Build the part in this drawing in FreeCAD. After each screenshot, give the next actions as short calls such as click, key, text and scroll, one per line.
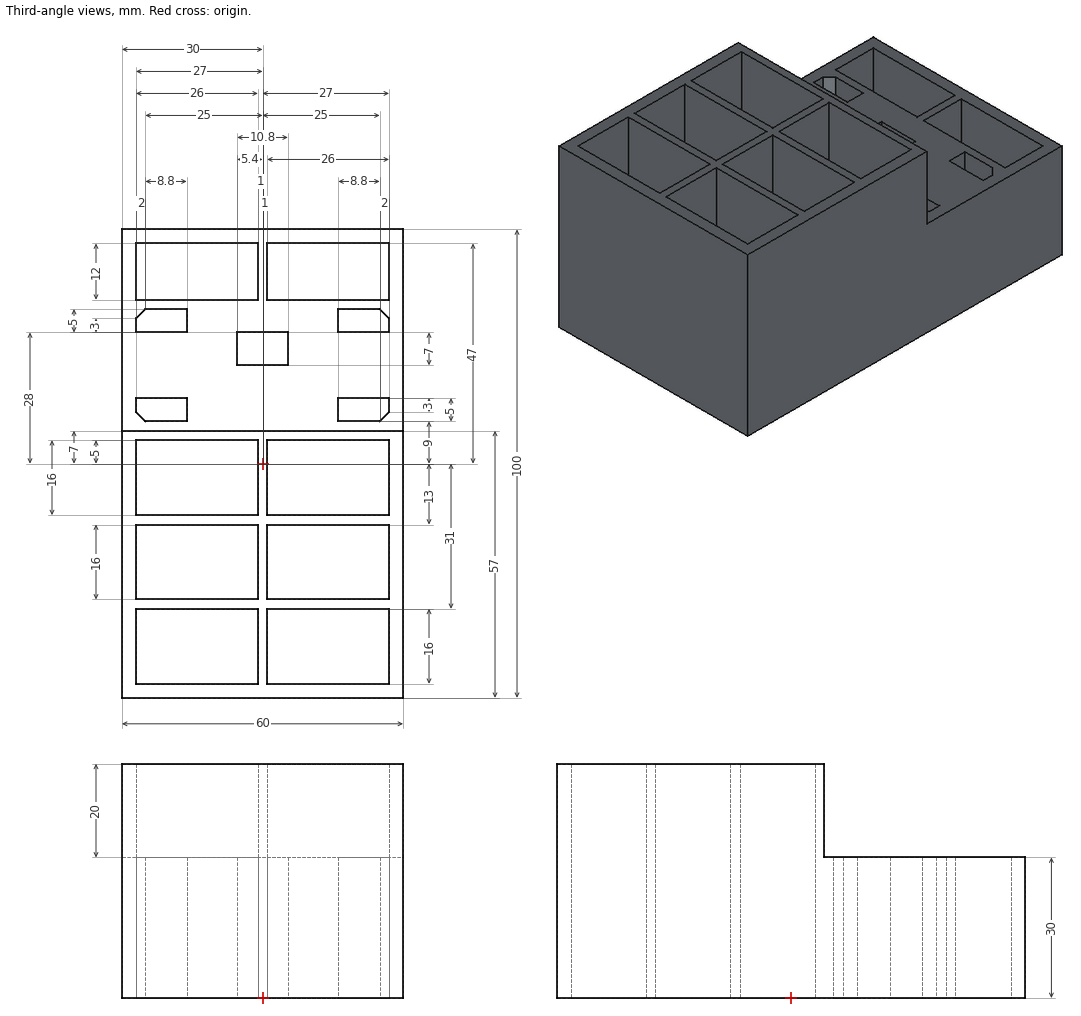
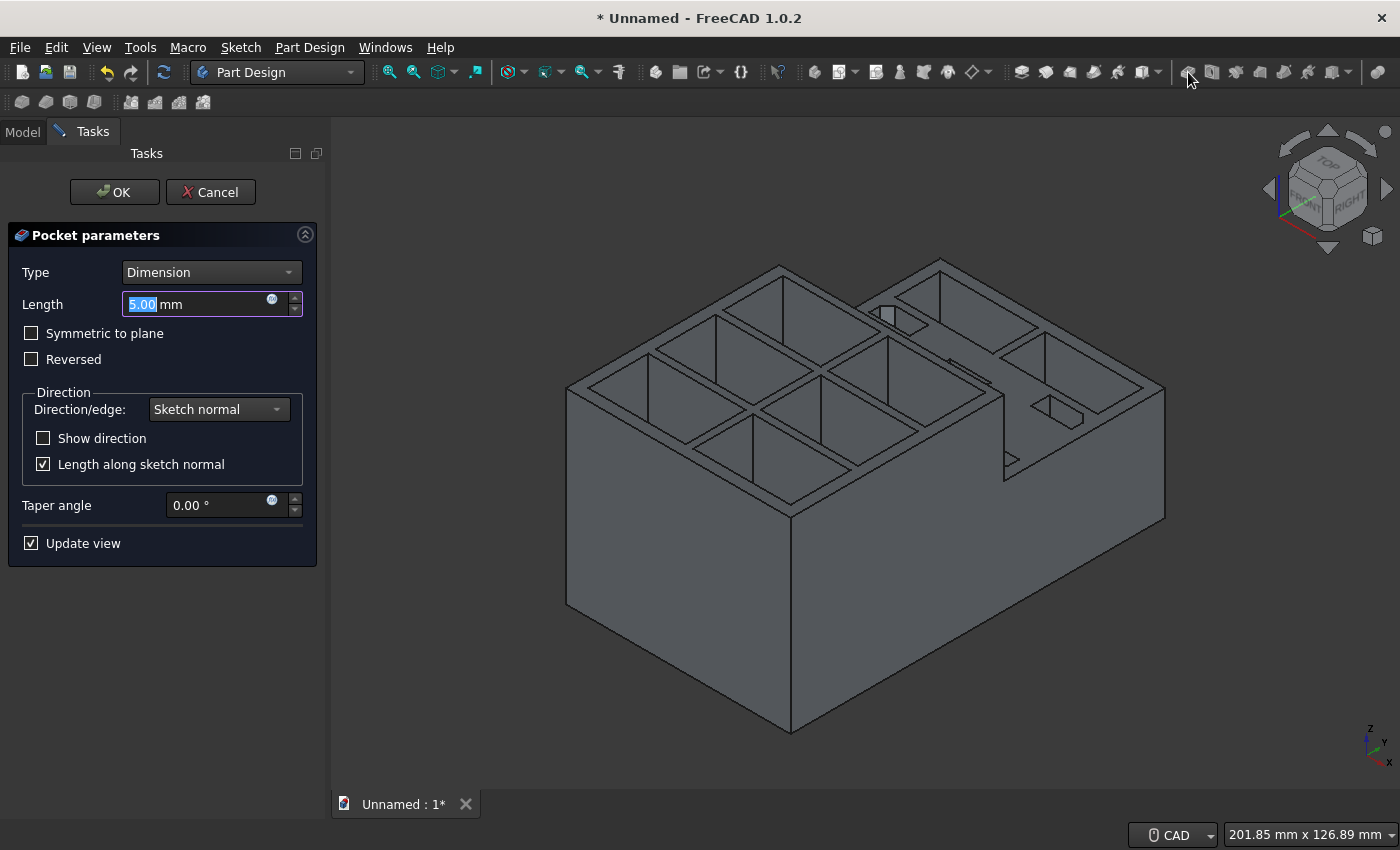
click(212, 272)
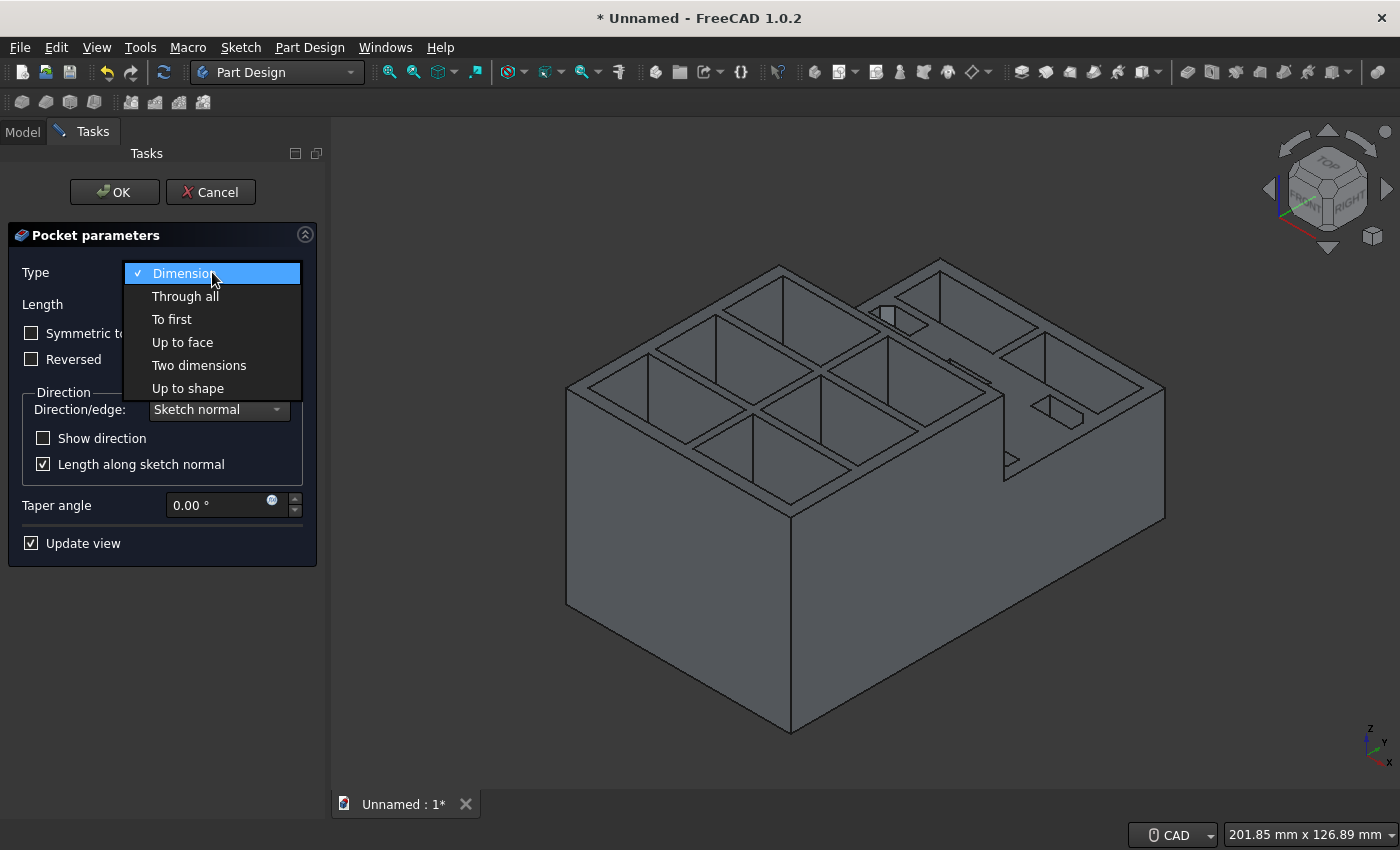
click(212, 296)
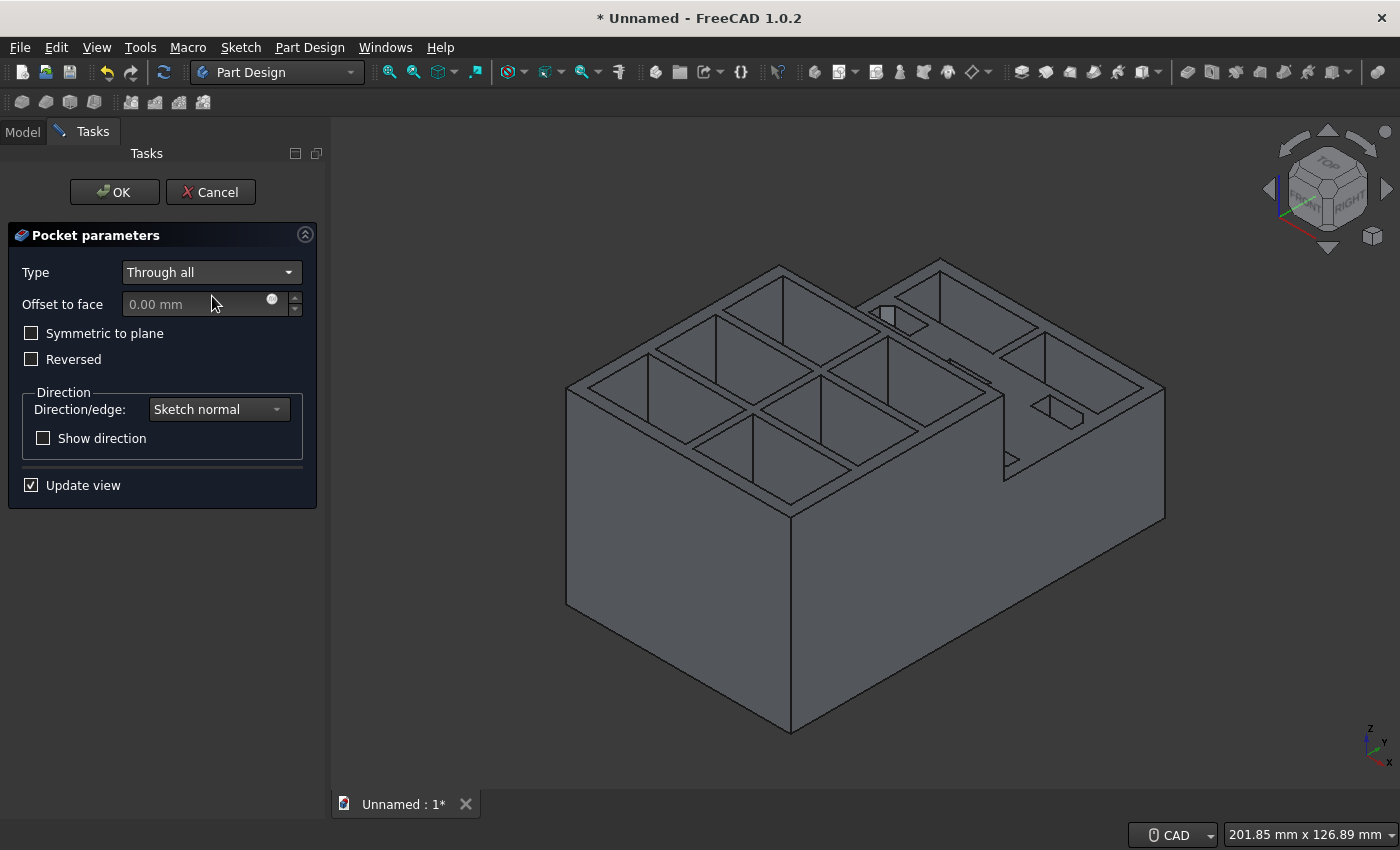
click(115, 192)